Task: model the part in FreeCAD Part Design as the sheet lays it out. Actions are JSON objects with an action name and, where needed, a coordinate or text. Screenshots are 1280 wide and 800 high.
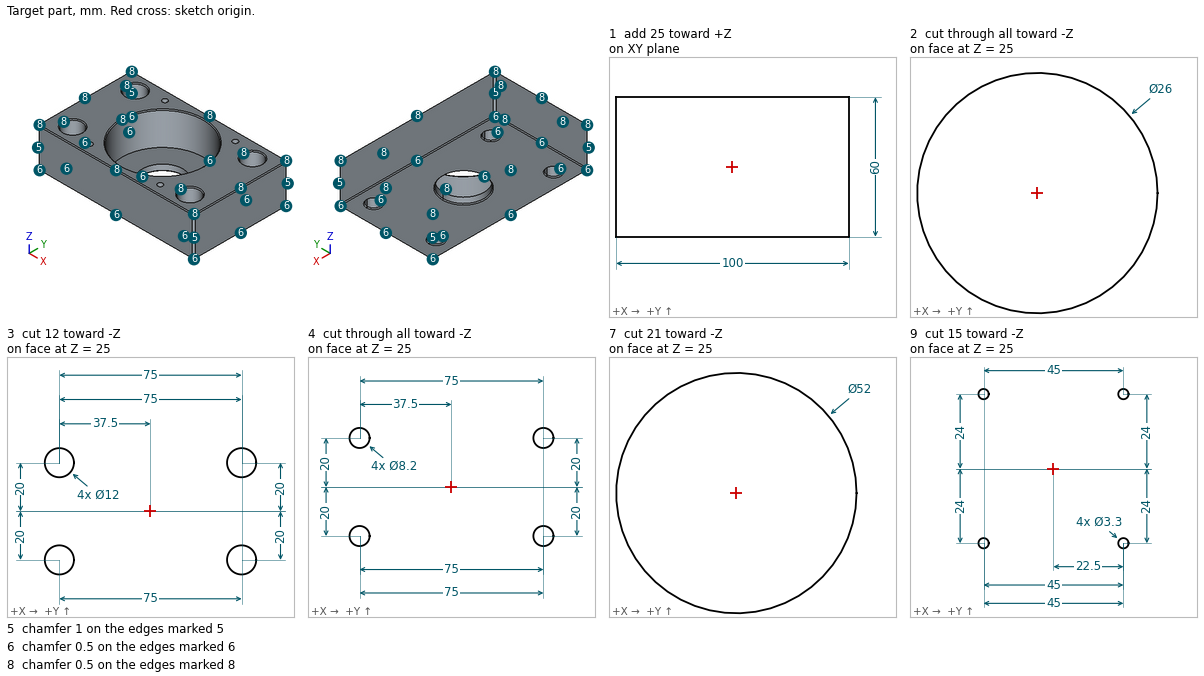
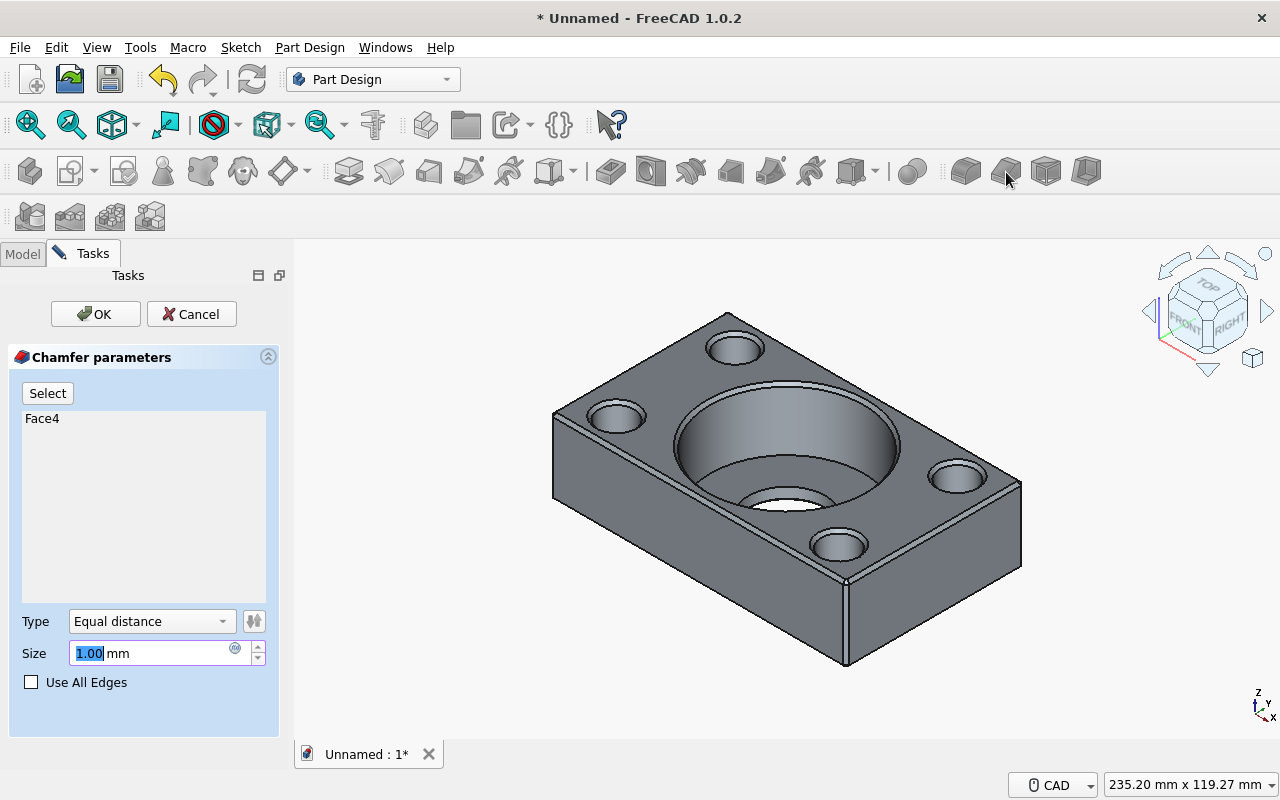
{"action": "type", "text": "0.5"}
{"action": "key", "text": "Tab"}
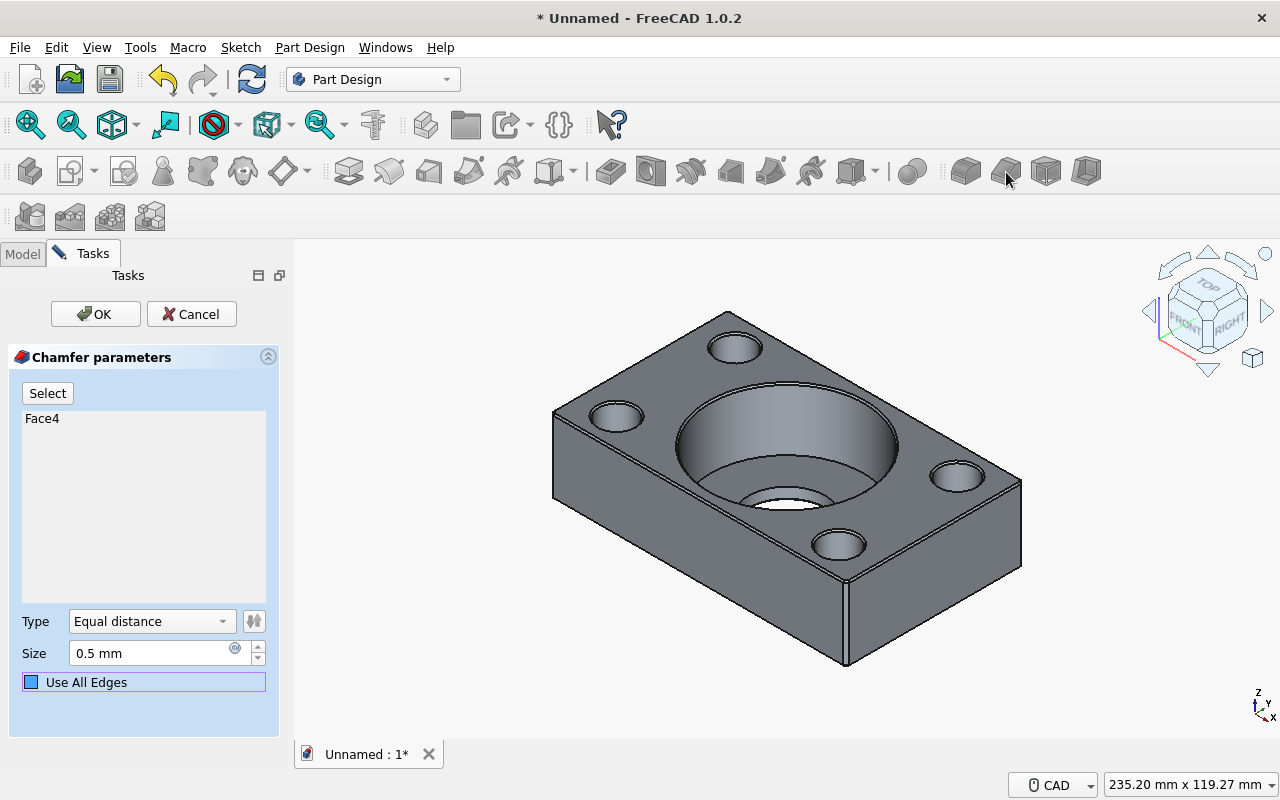
{"action": "left_click", "coordinate": [96, 314]}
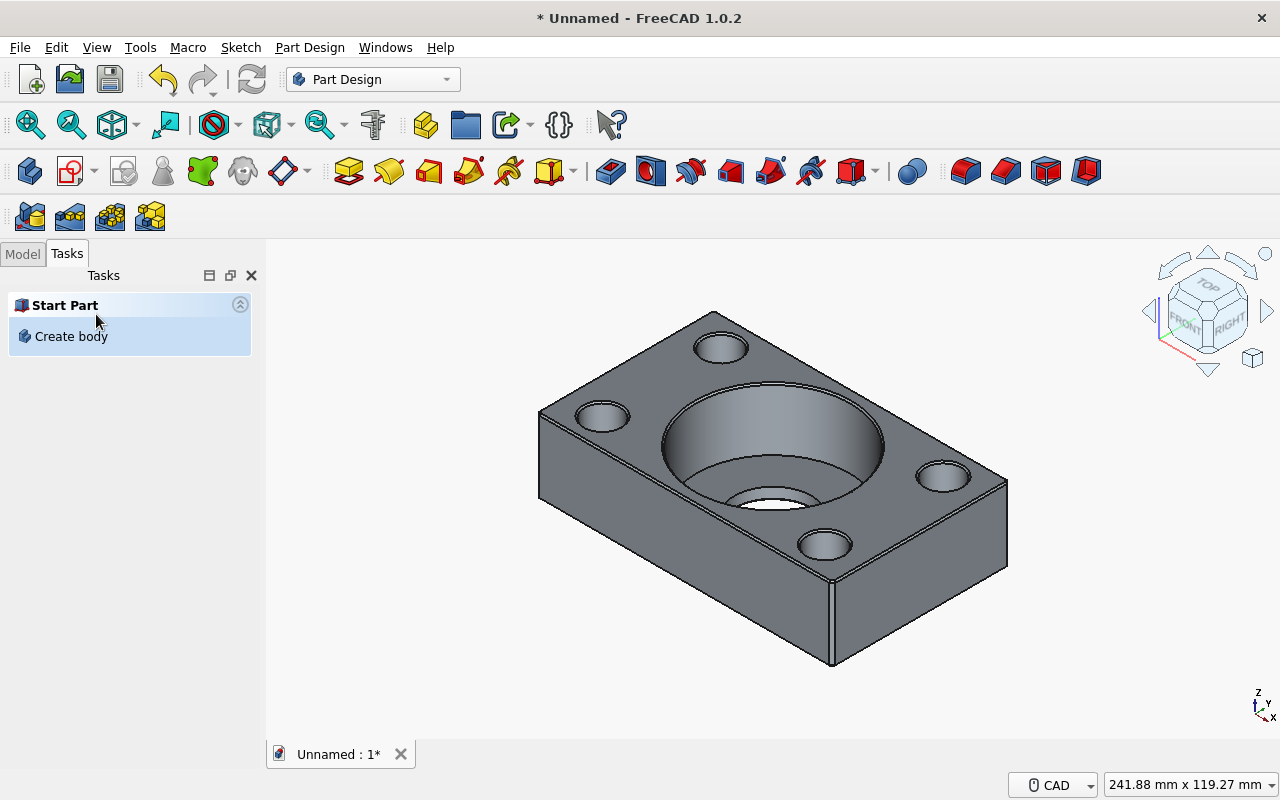
{"action": "left_click", "coordinate": [899, 518]}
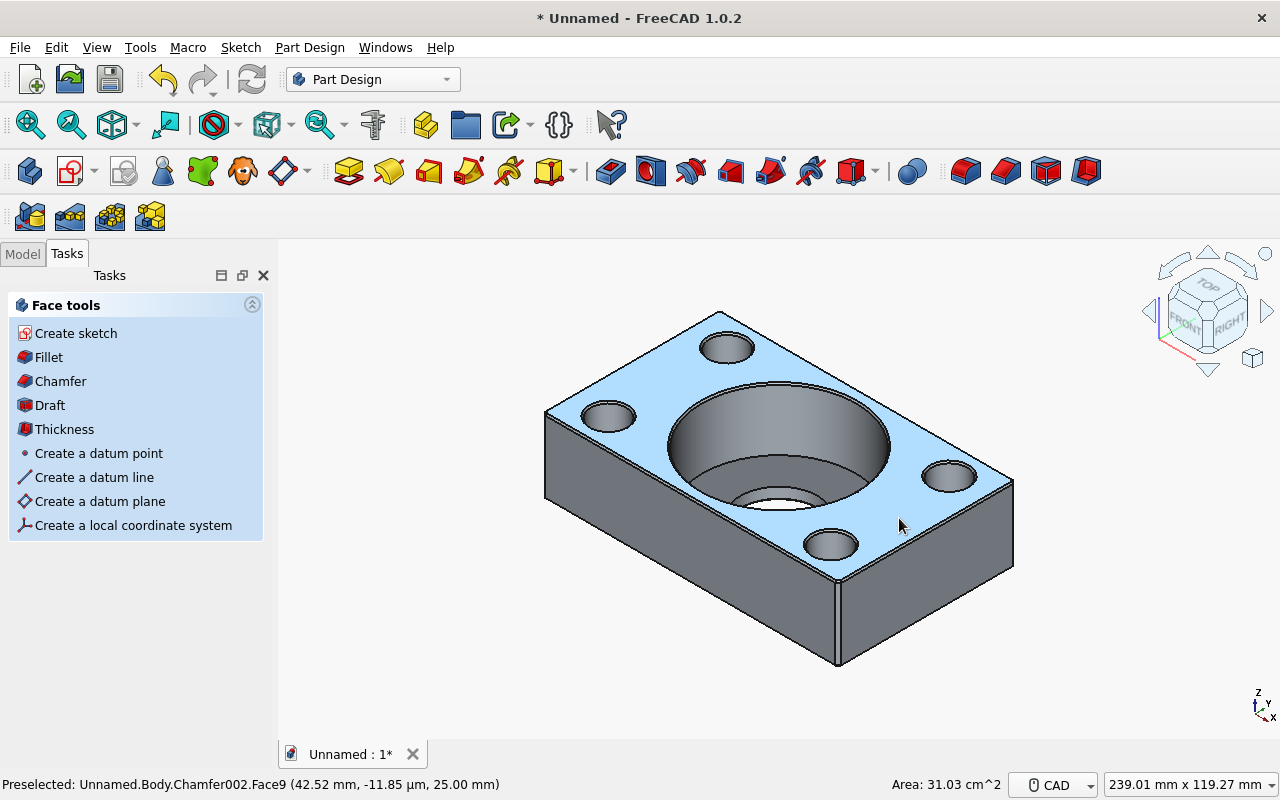
{"action": "left_click", "coordinate": [70, 172]}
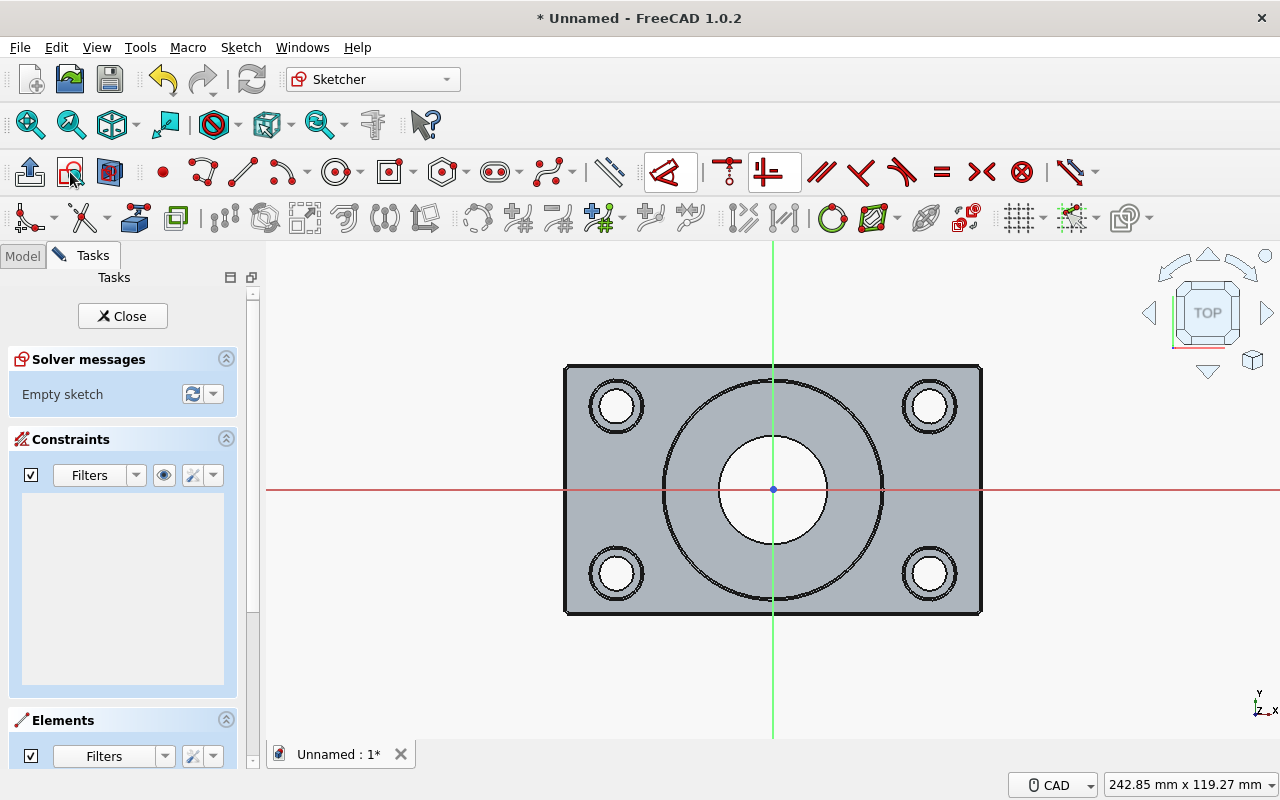
{"action": "scroll", "coordinate": [912, 490], "scroll_direction": "up", "scroll_amount": 2}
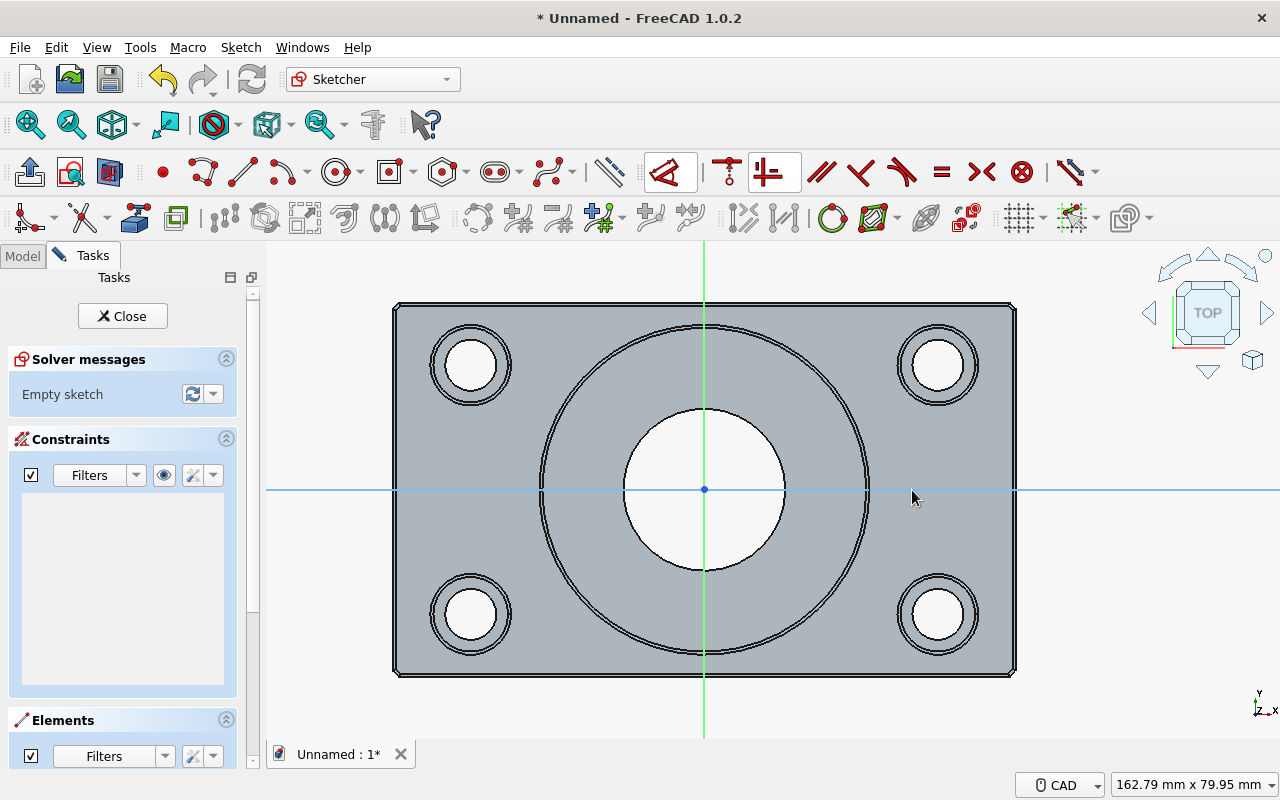
{"action": "key", "text": "g c"}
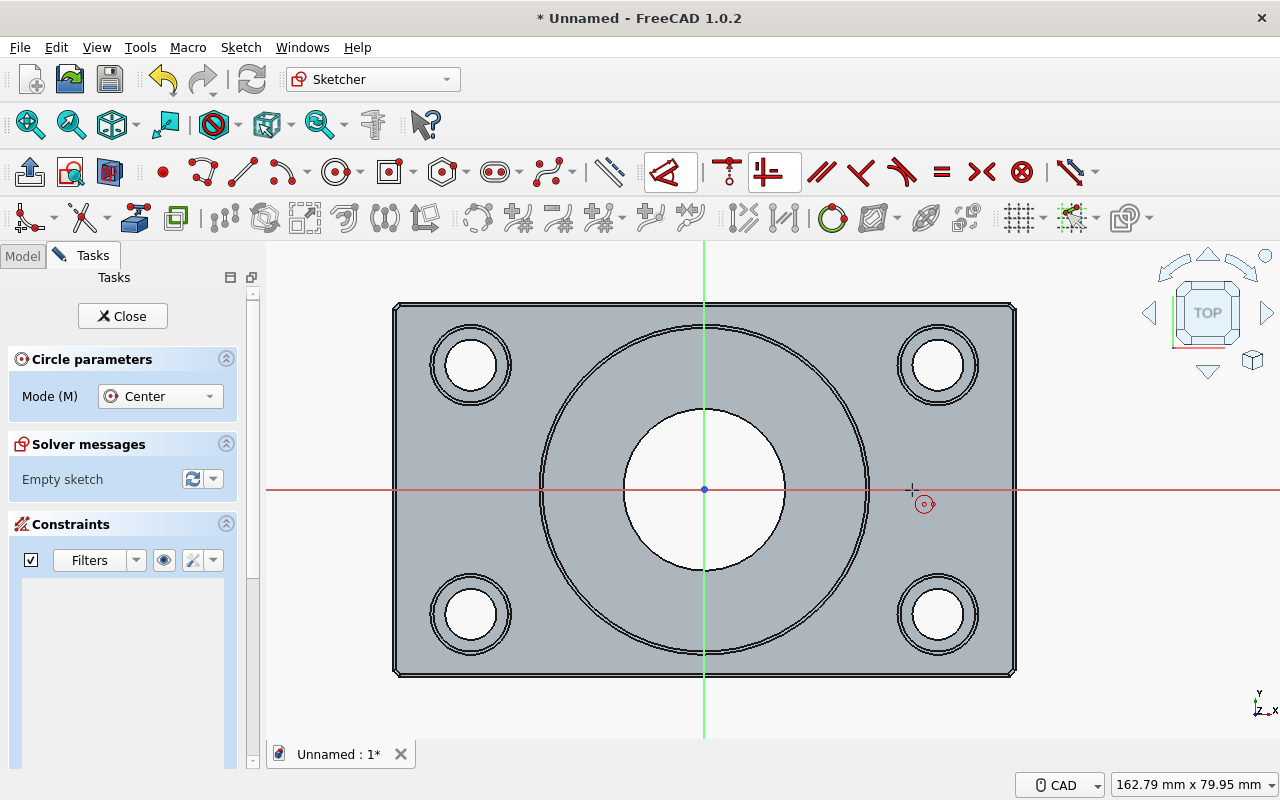
{"action": "scroll", "coordinate": [844, 639], "scroll_direction": "up", "scroll_amount": 4}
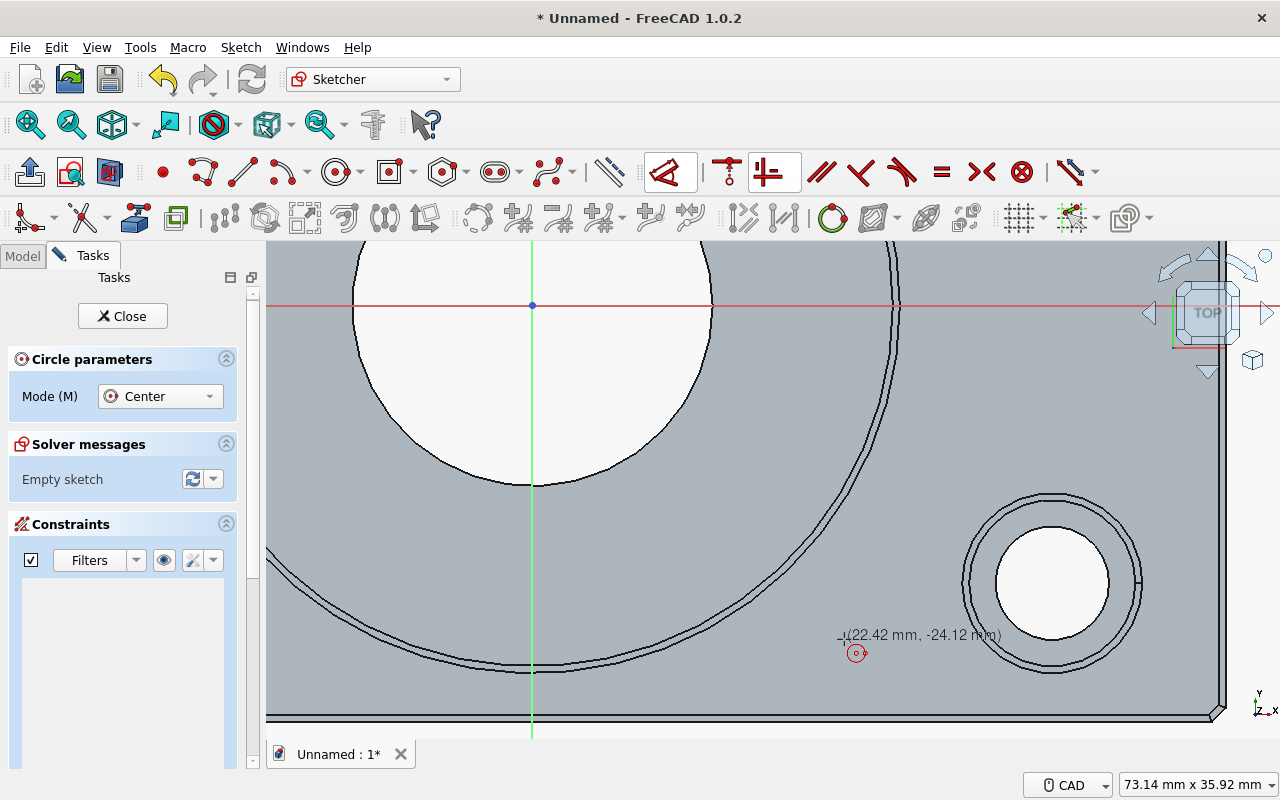
{"action": "left_click", "coordinate": [844, 639]}
{"action": "mouse_move", "coordinate": [861, 622]}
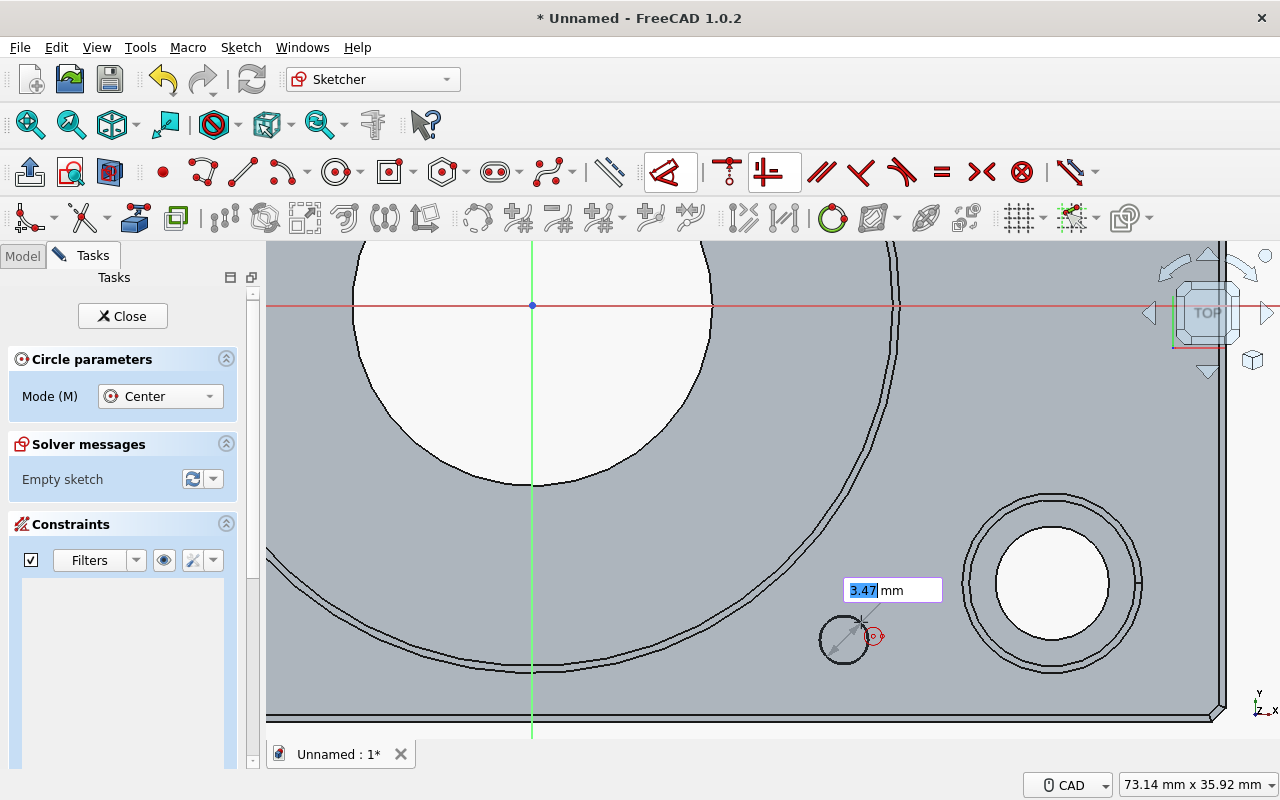
{"action": "type", "text": "3.3"}
{"action": "key", "text": "Return"}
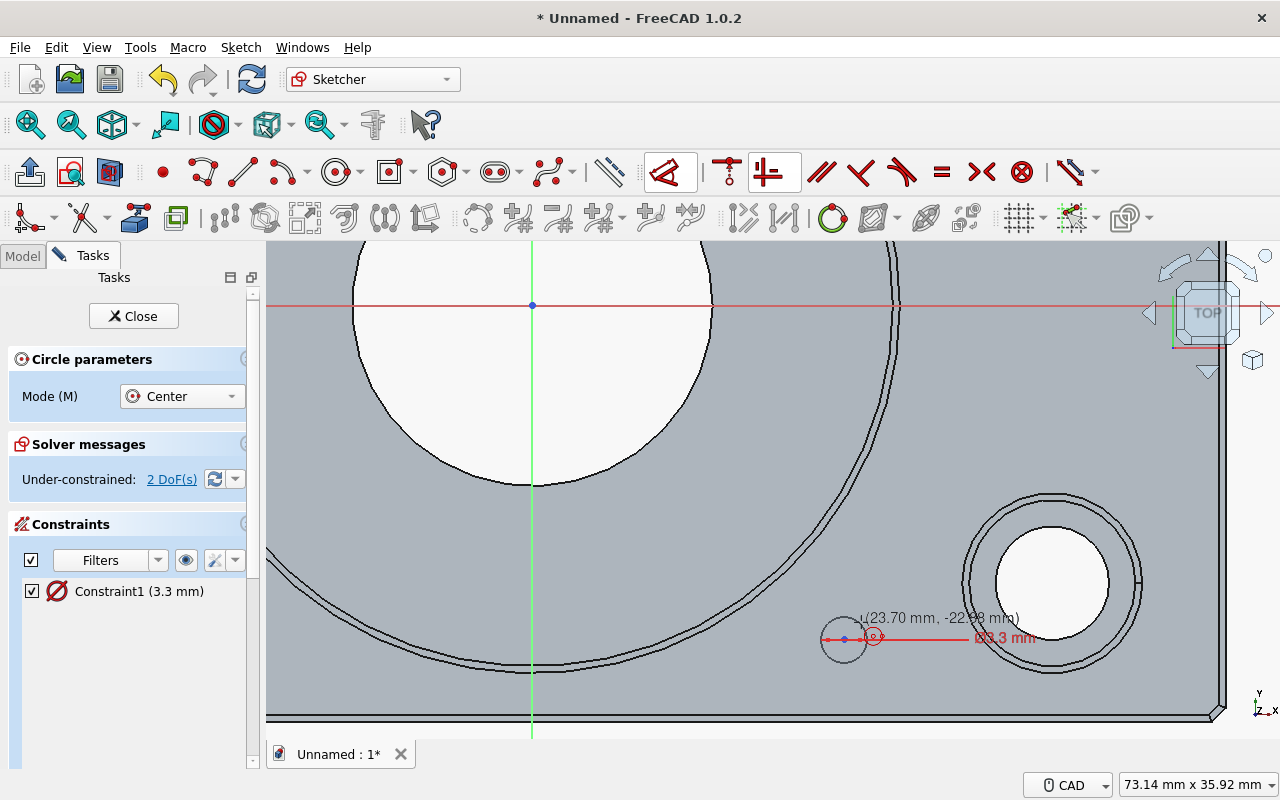
{"action": "scroll", "coordinate": [845, 640], "scroll_direction": "down", "scroll_amount": 4}